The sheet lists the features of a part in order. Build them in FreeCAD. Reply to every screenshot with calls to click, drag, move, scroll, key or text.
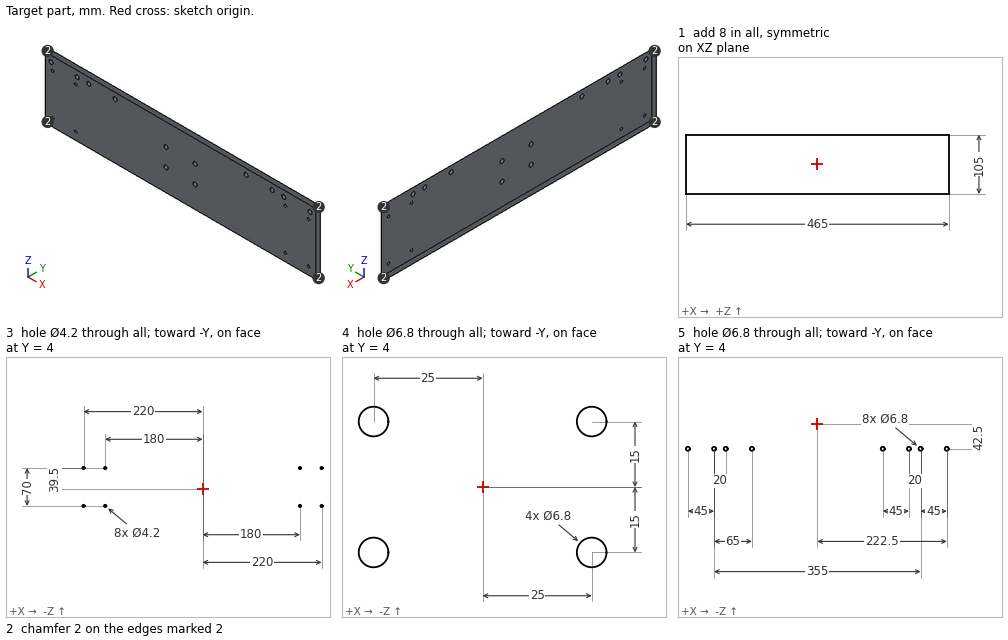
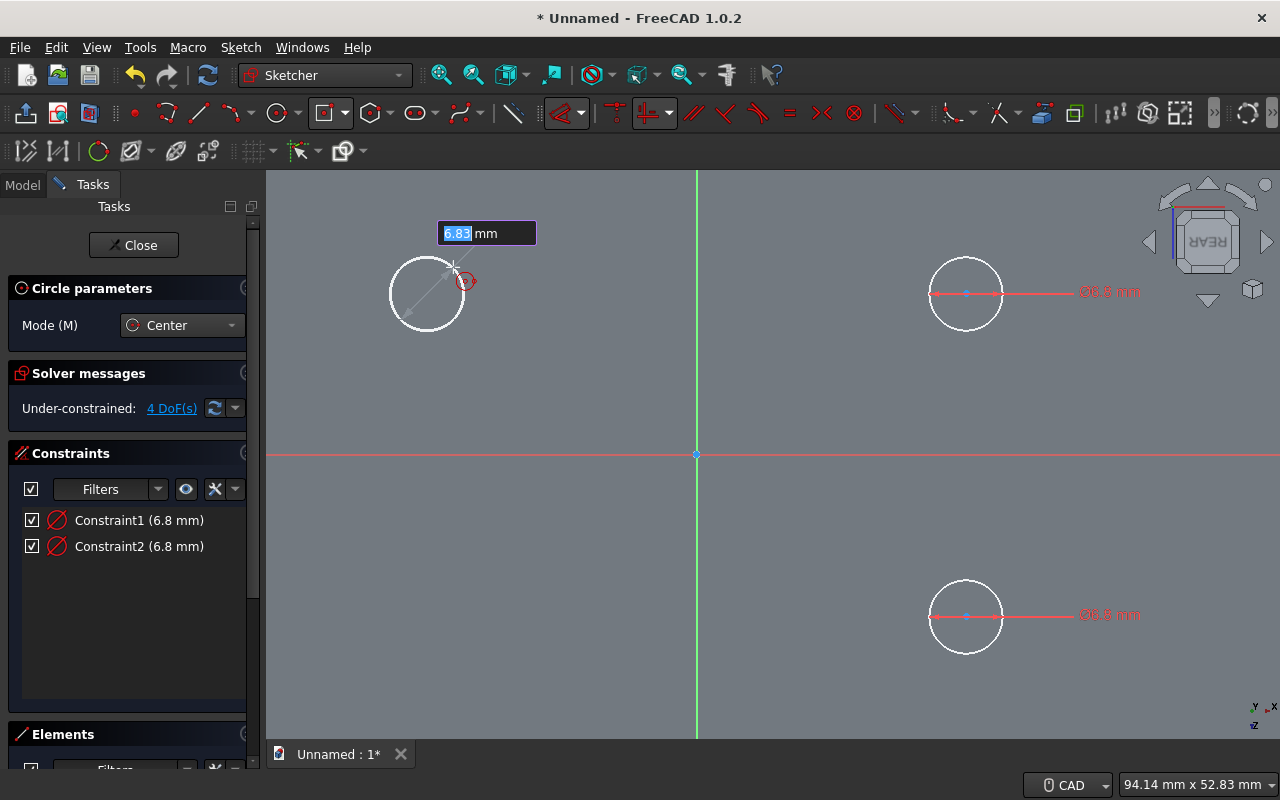
text(6.8)
key(Return)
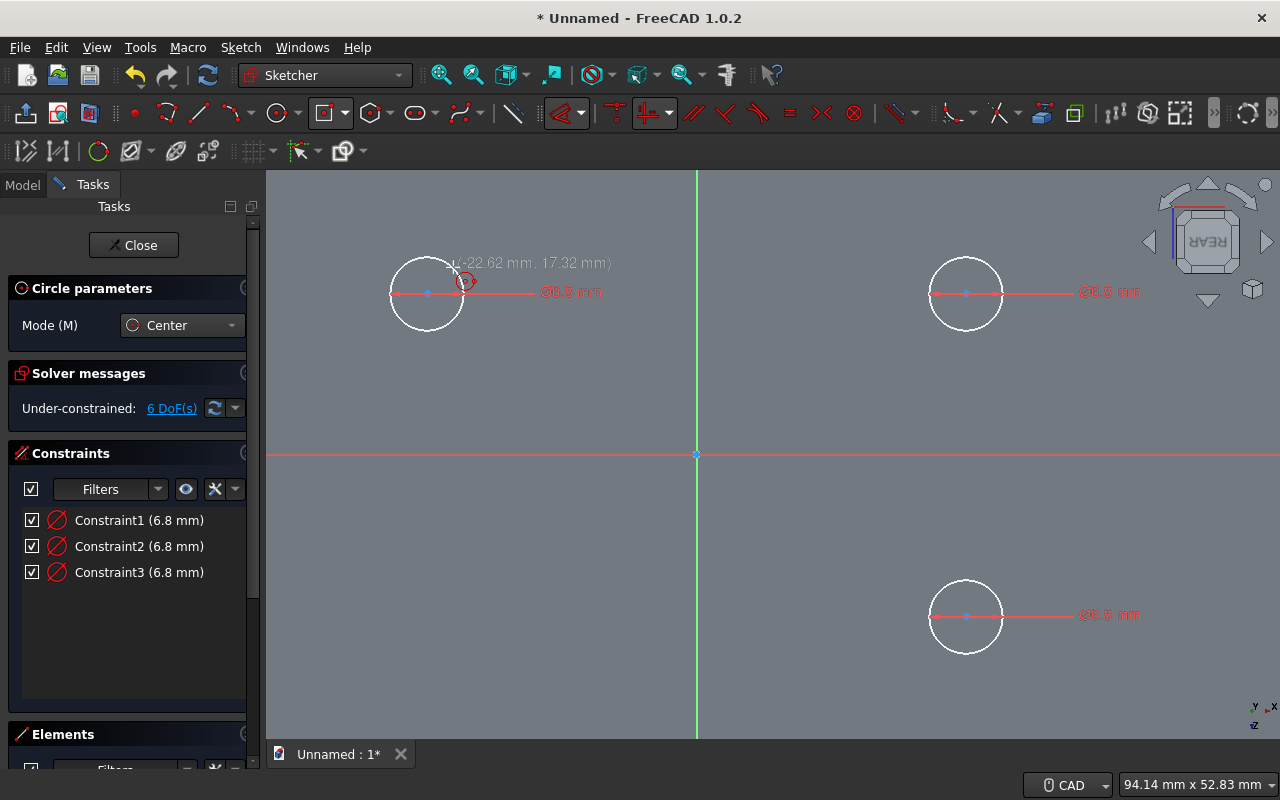
click(427, 616)
move(453, 590)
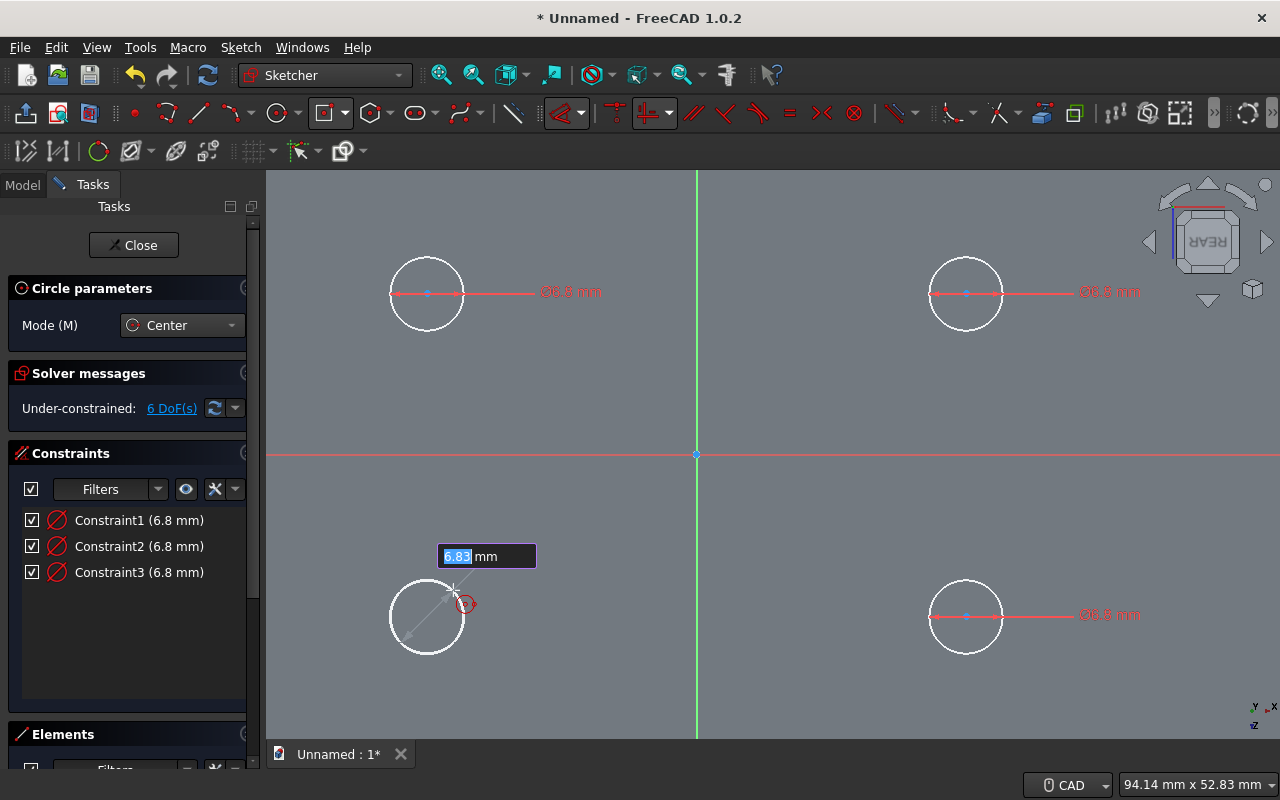
text(6.8)
key(Return)
key(Escape)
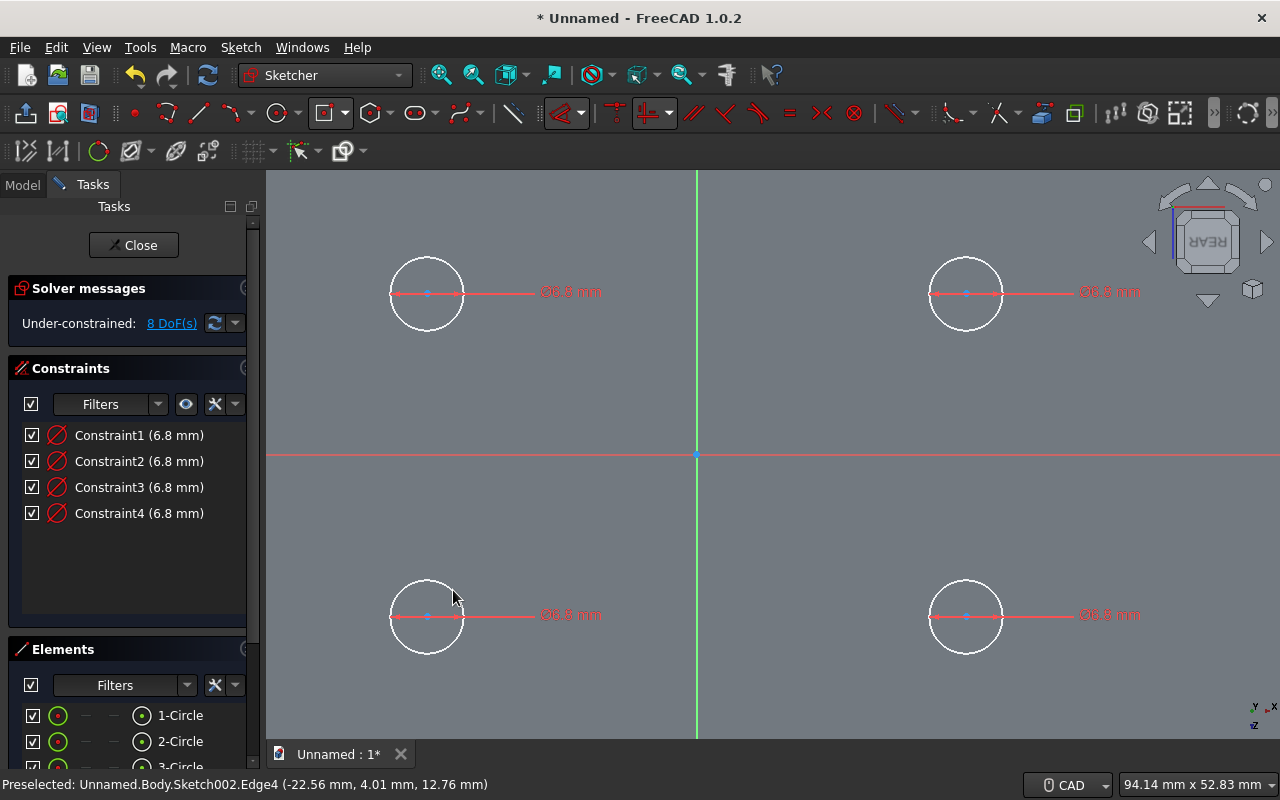
click(966, 617)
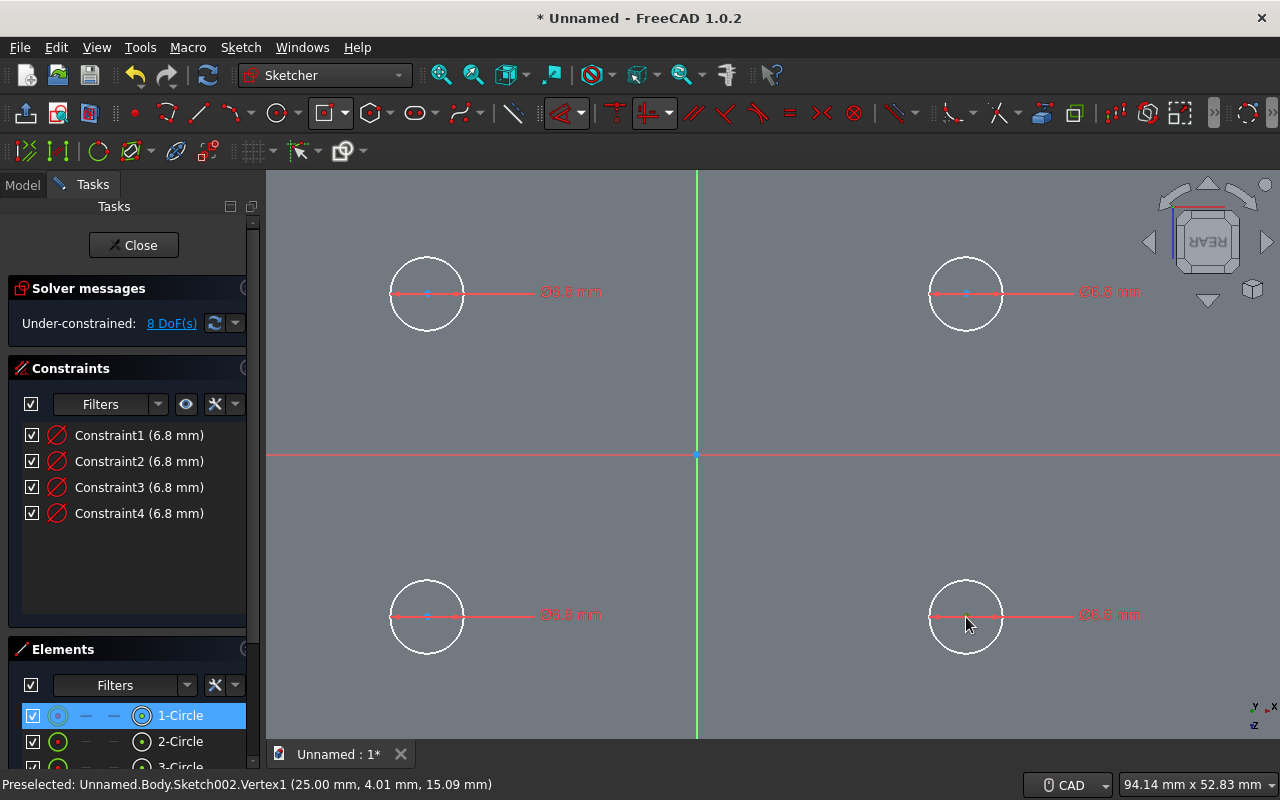
click(966, 294)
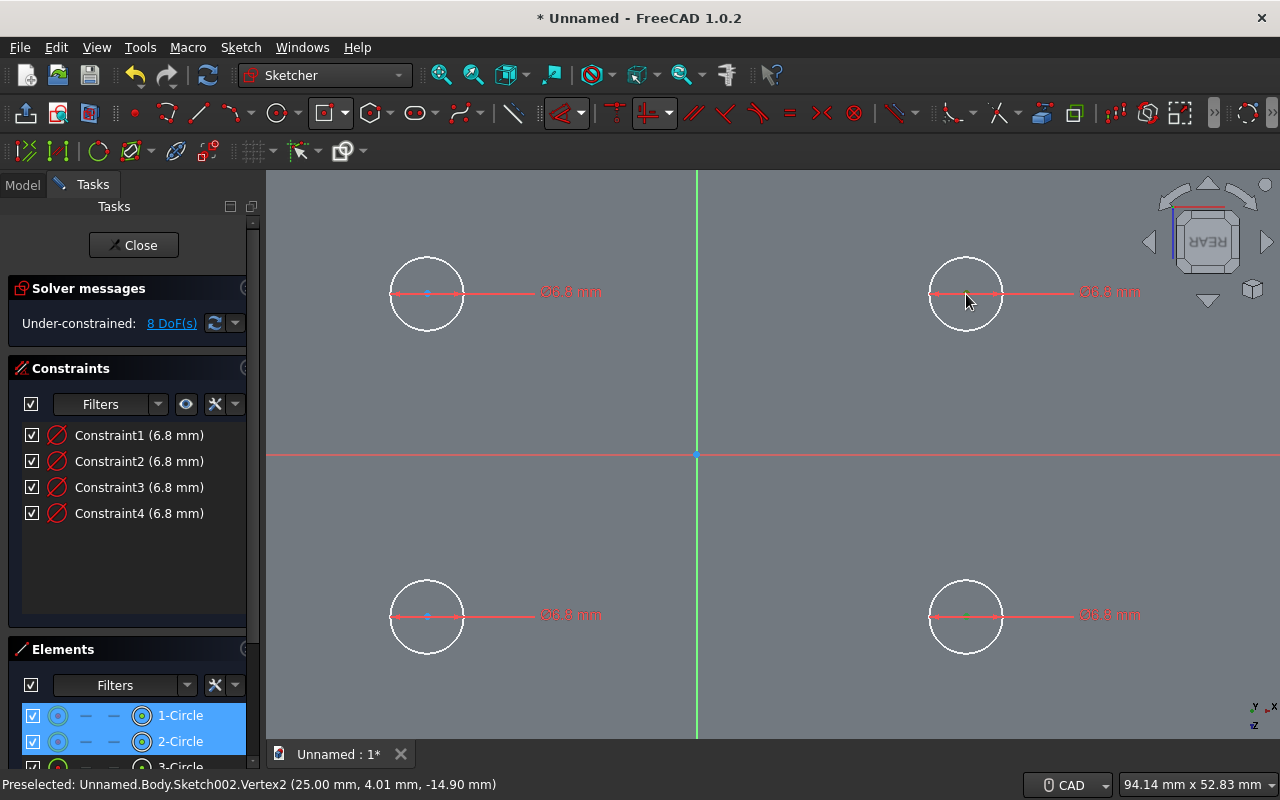
click(672, 114)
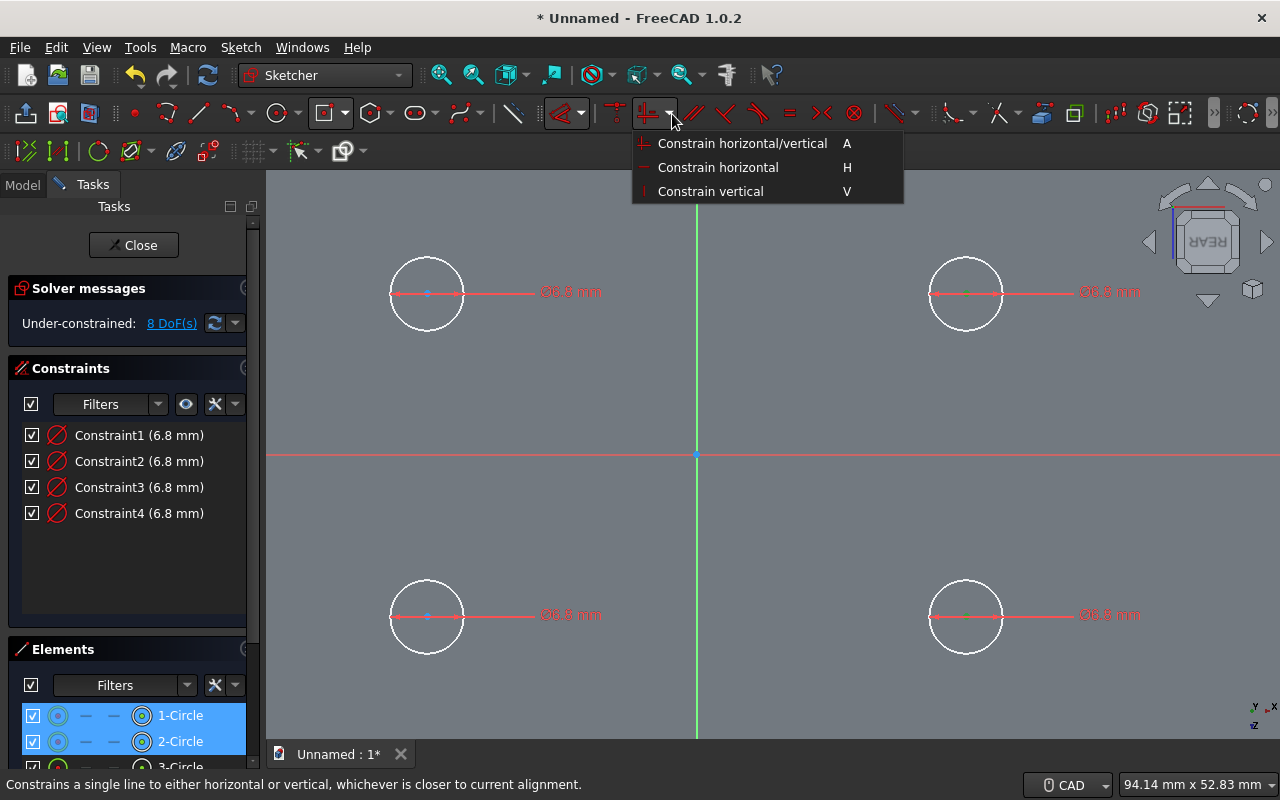
click(768, 191)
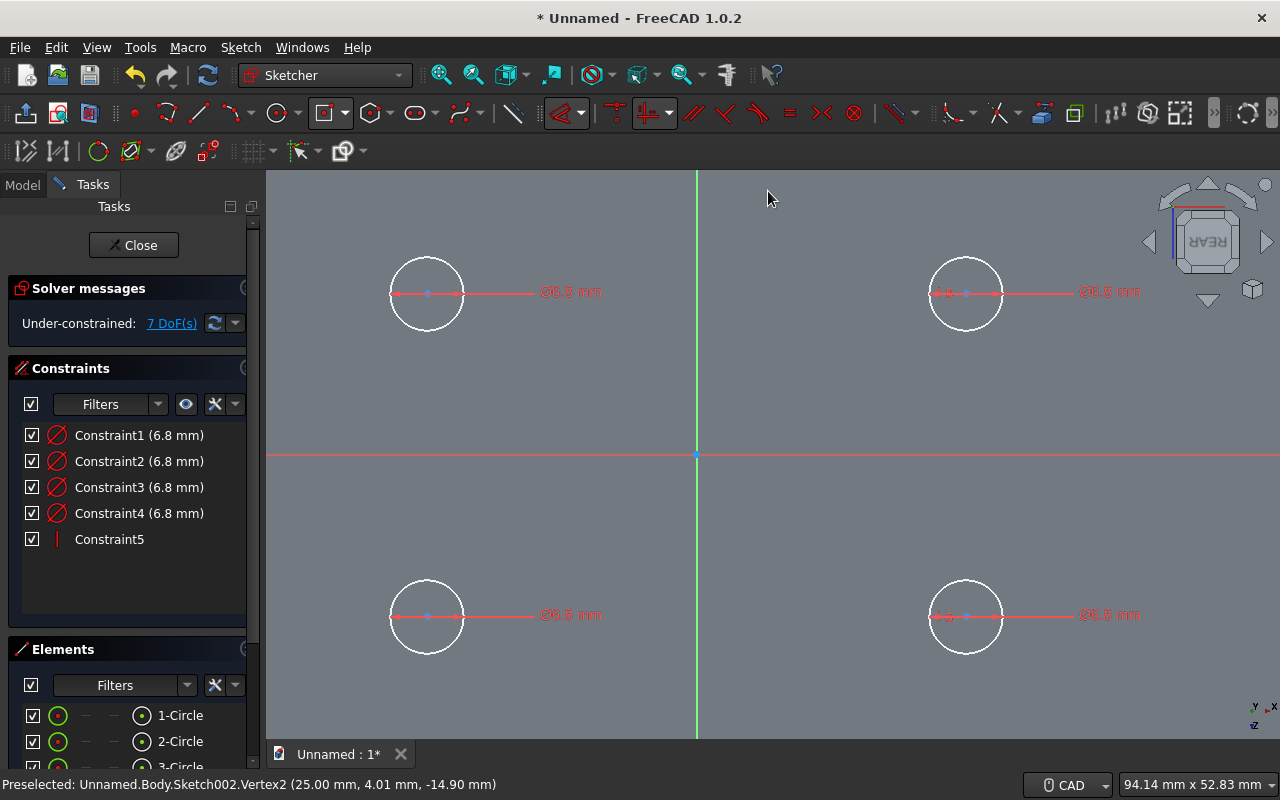
click(966, 294)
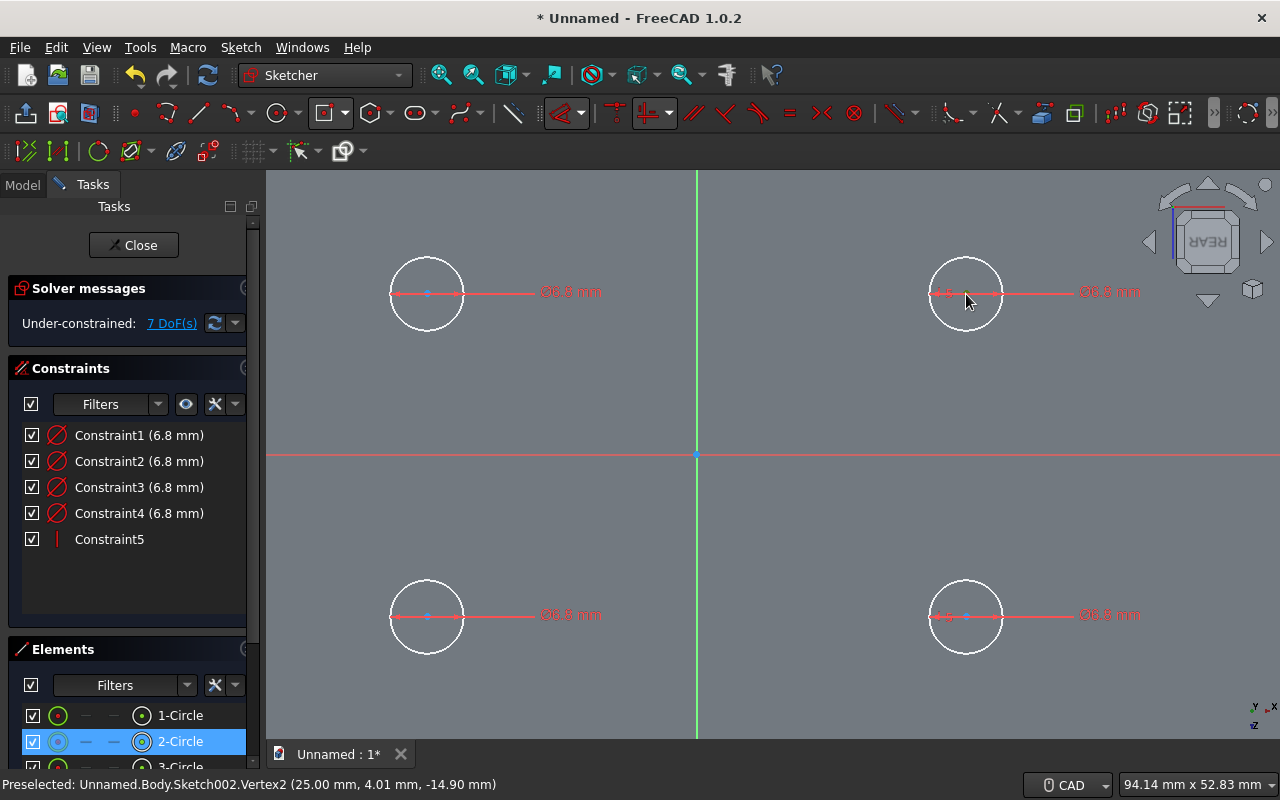
click(427, 294)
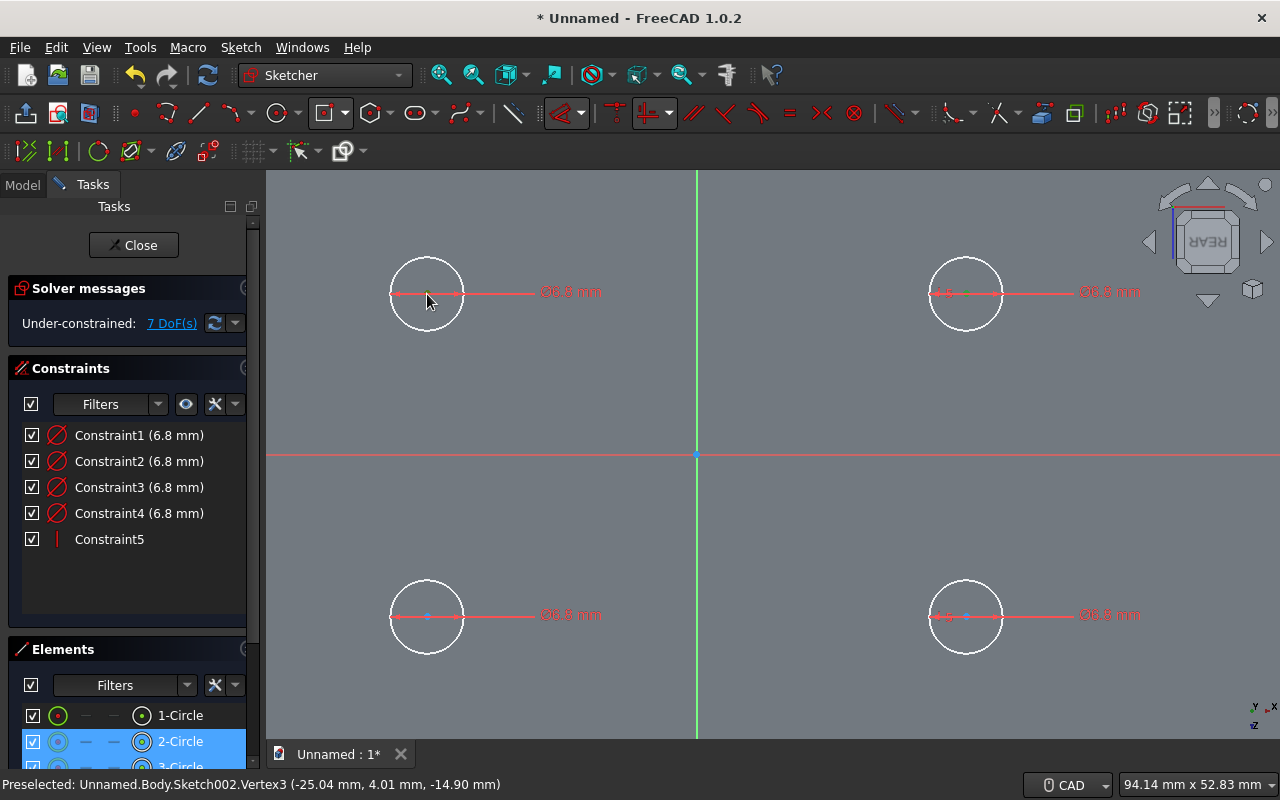
click(672, 114)